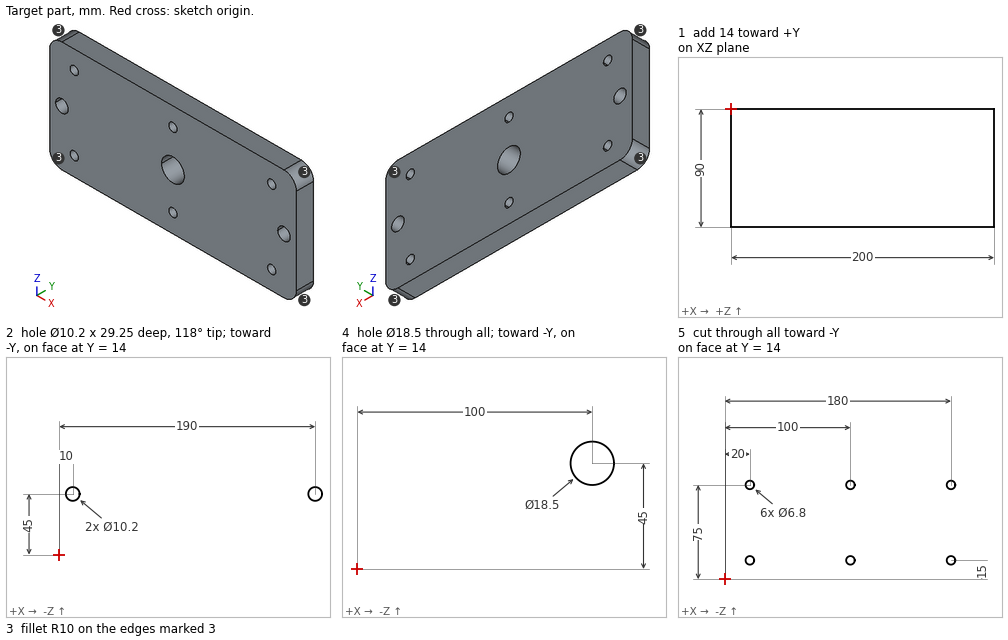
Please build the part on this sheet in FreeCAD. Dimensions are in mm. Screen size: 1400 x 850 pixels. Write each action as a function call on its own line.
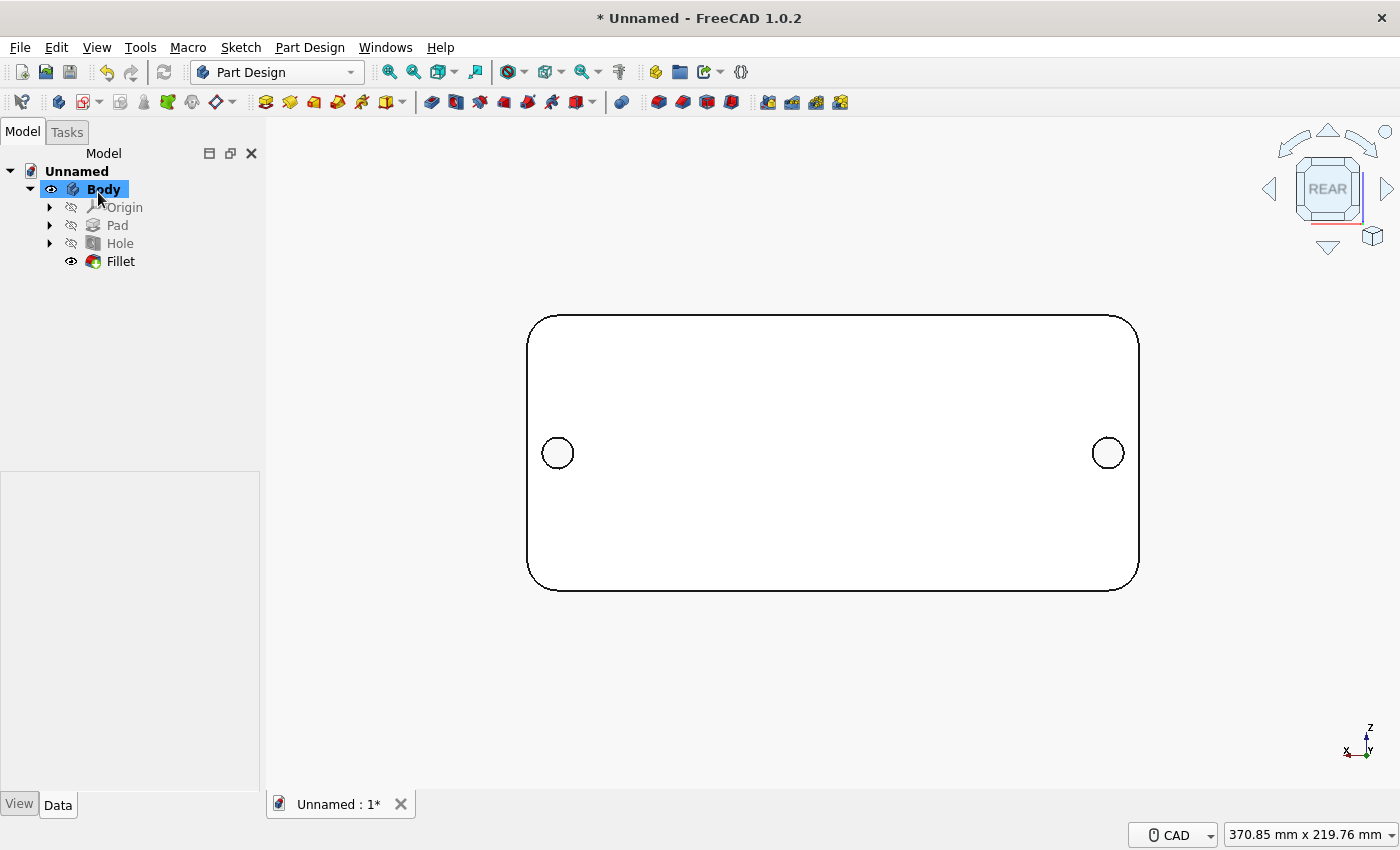
click(746, 452)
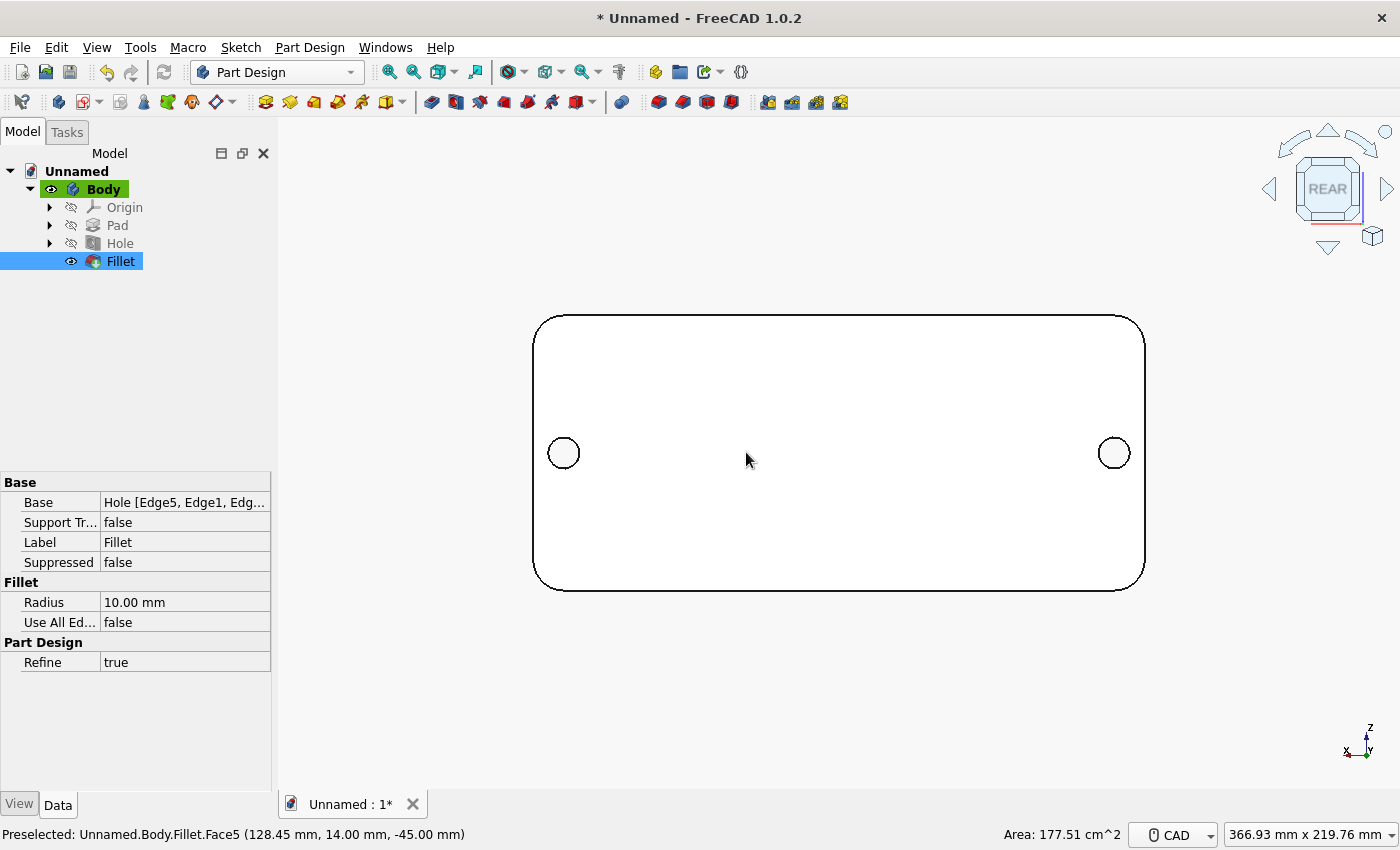
click(84, 102)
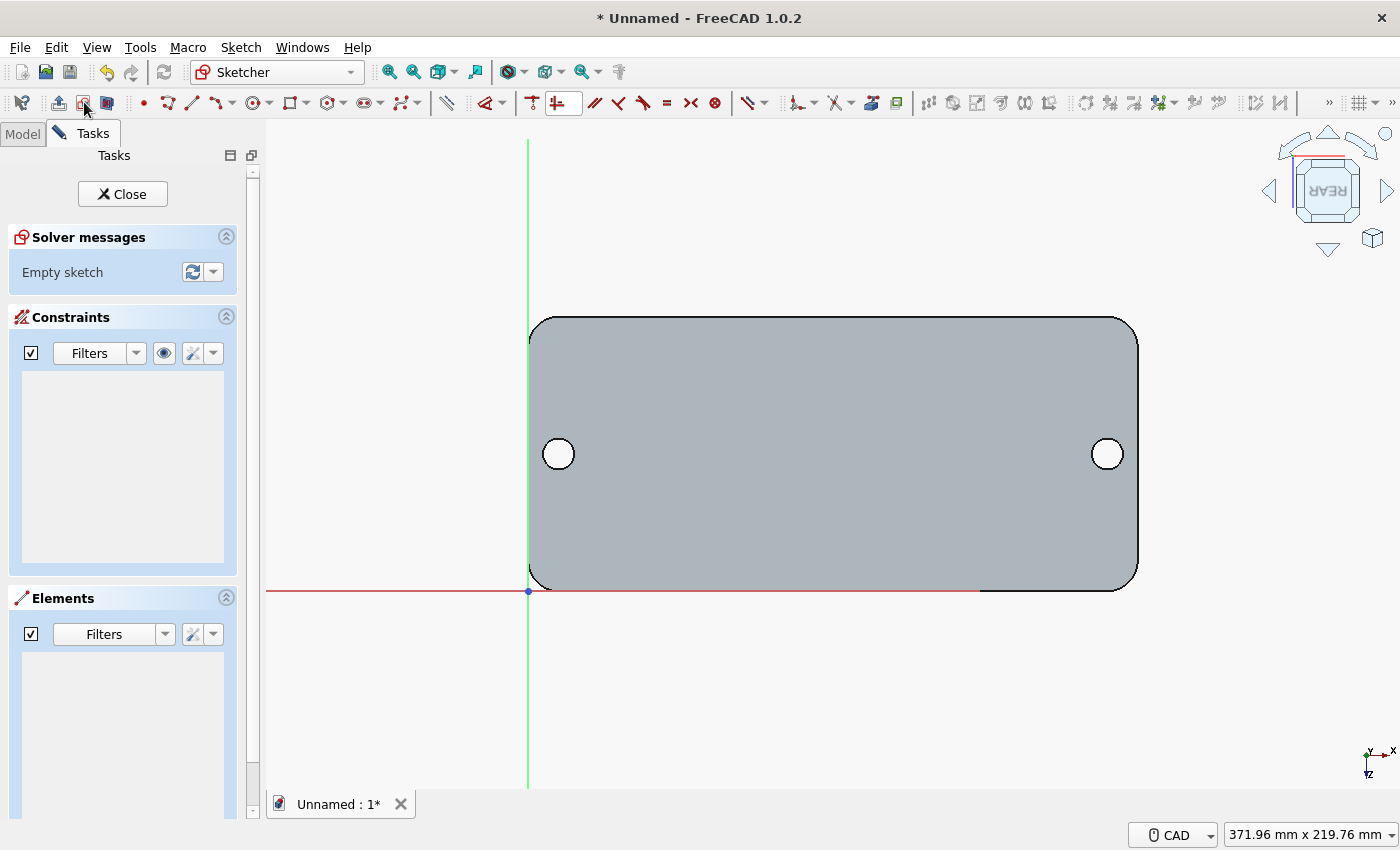
scroll(844, 454, up, 10)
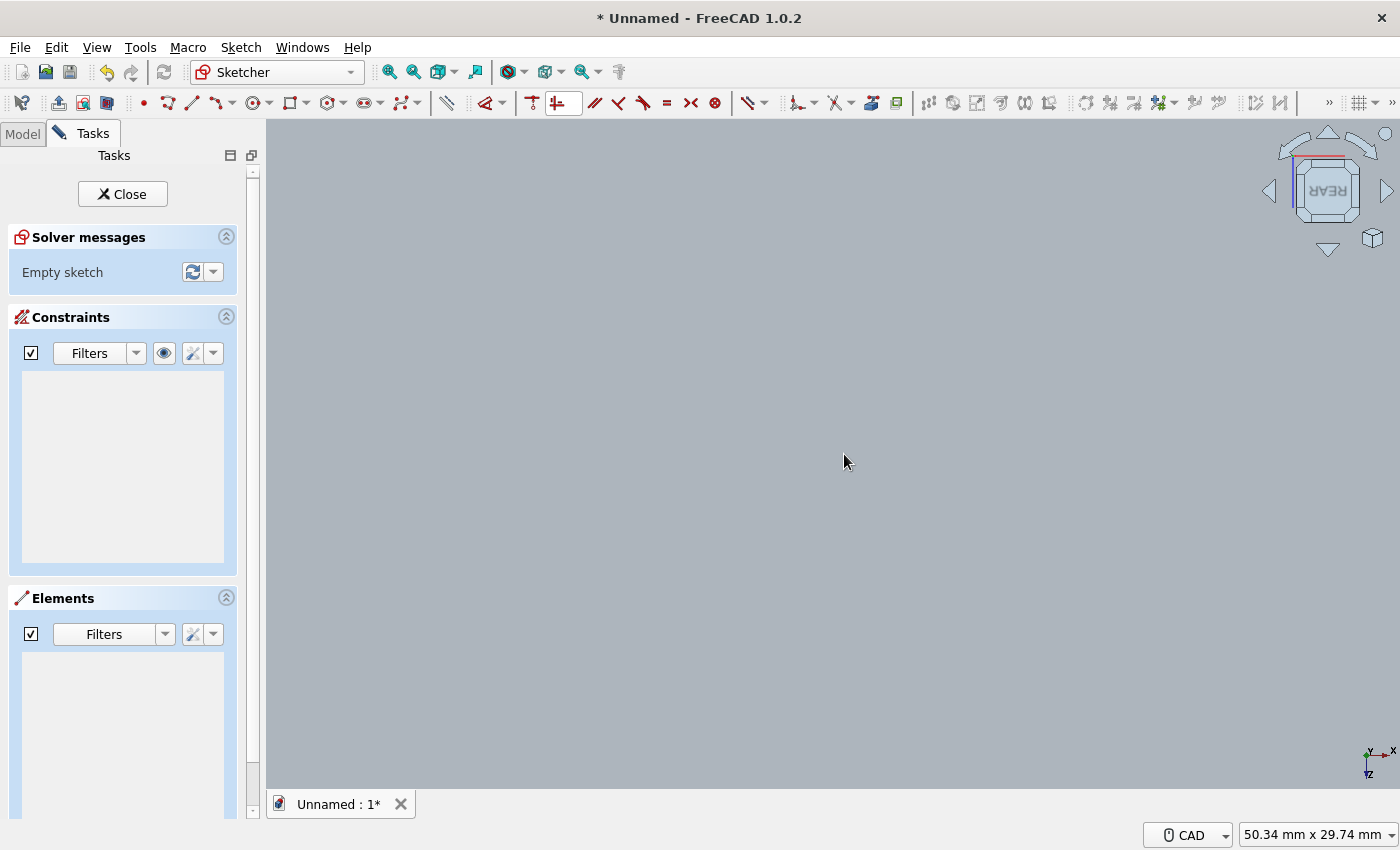
click(254, 104)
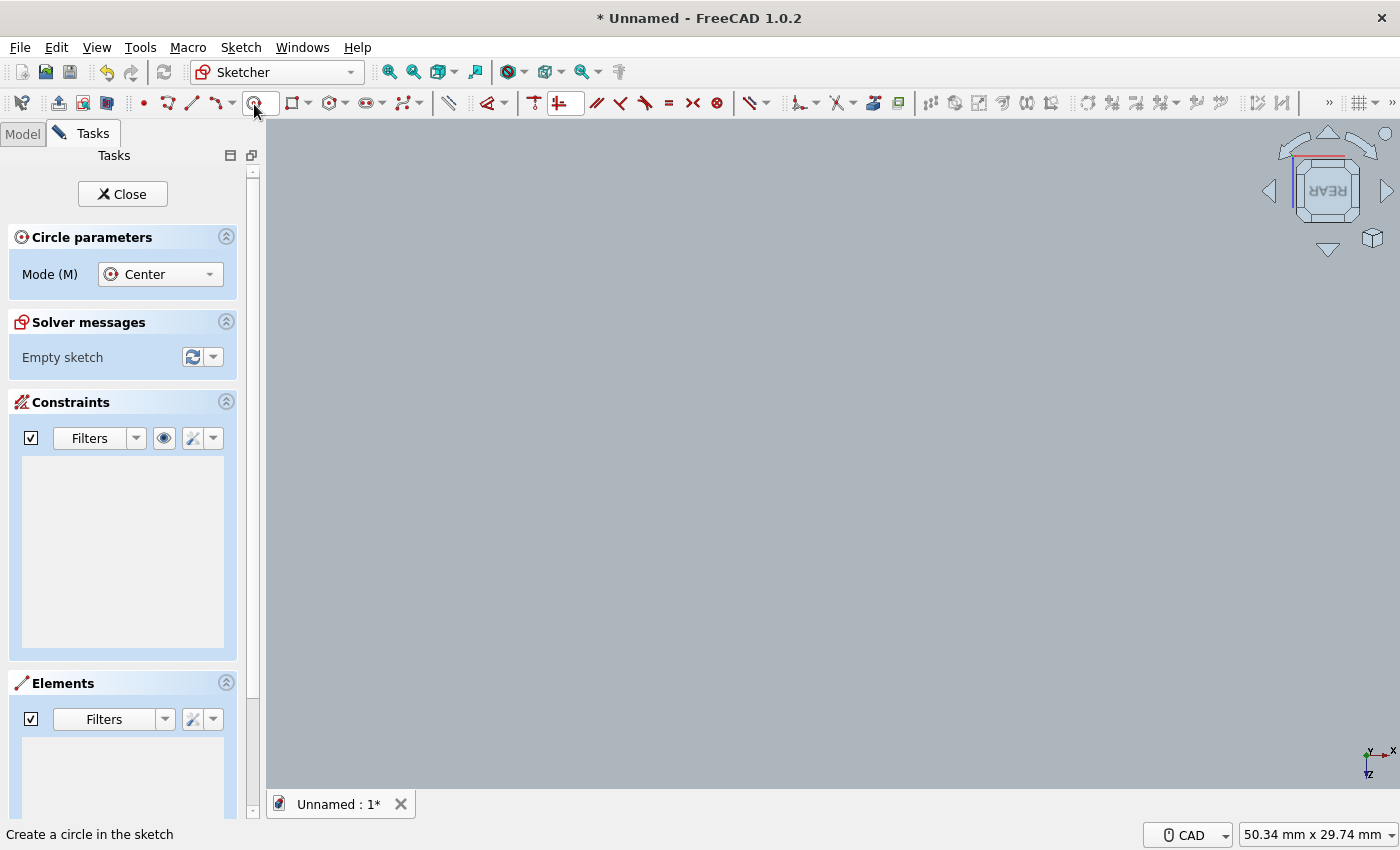
click(759, 451)
click(907, 303)
key(Escape)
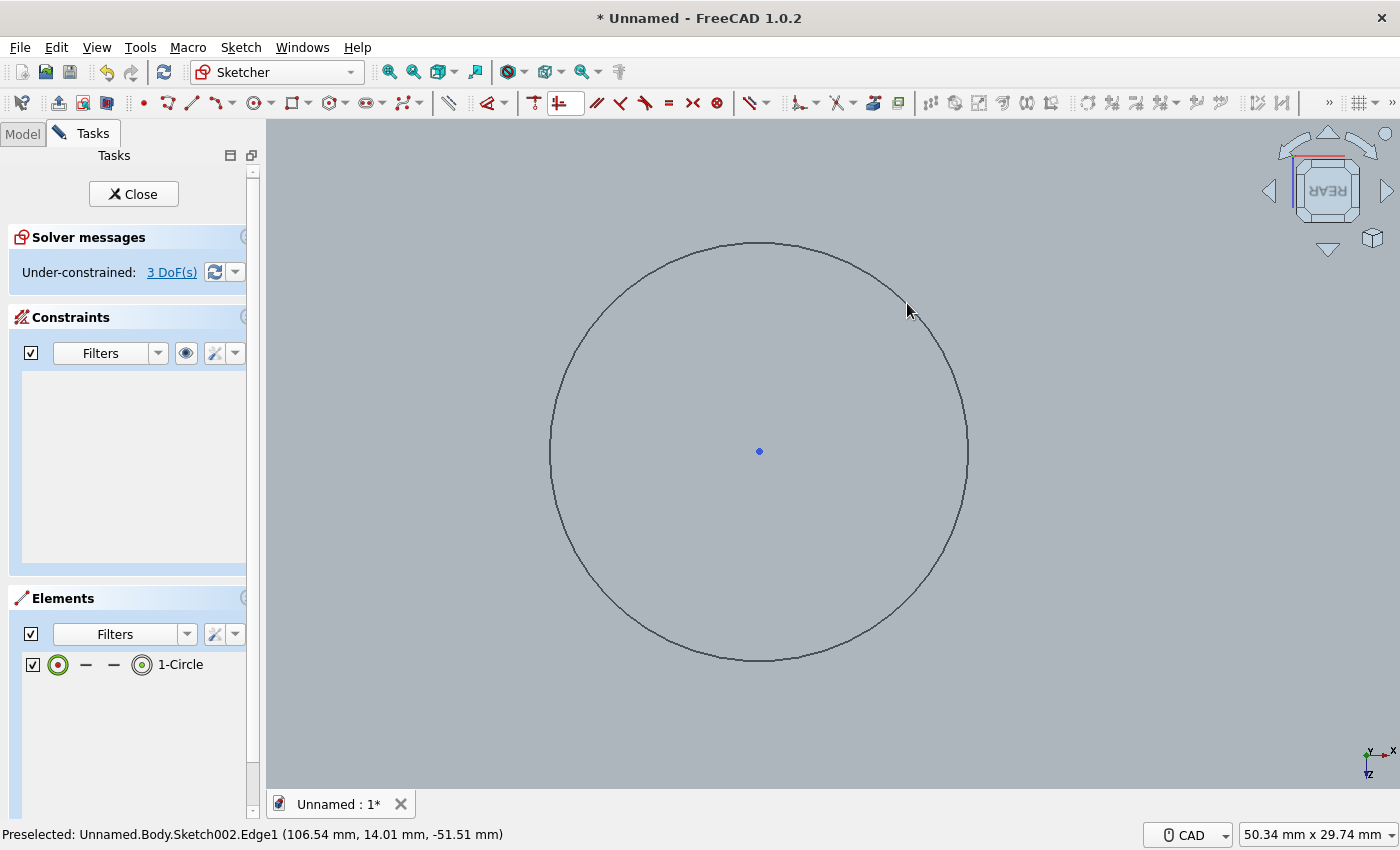
click(488, 104)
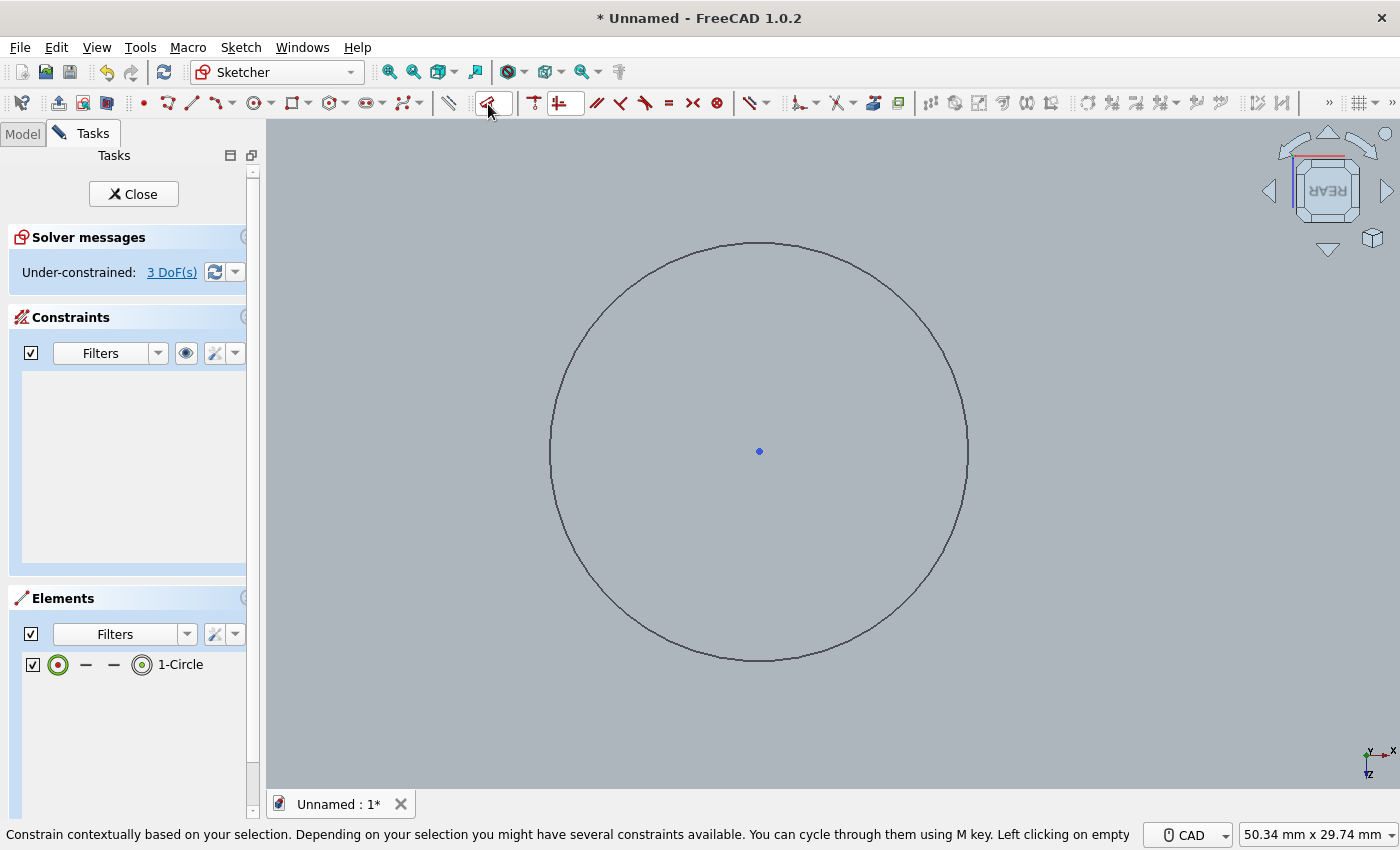
click(907, 304)
click(930, 281)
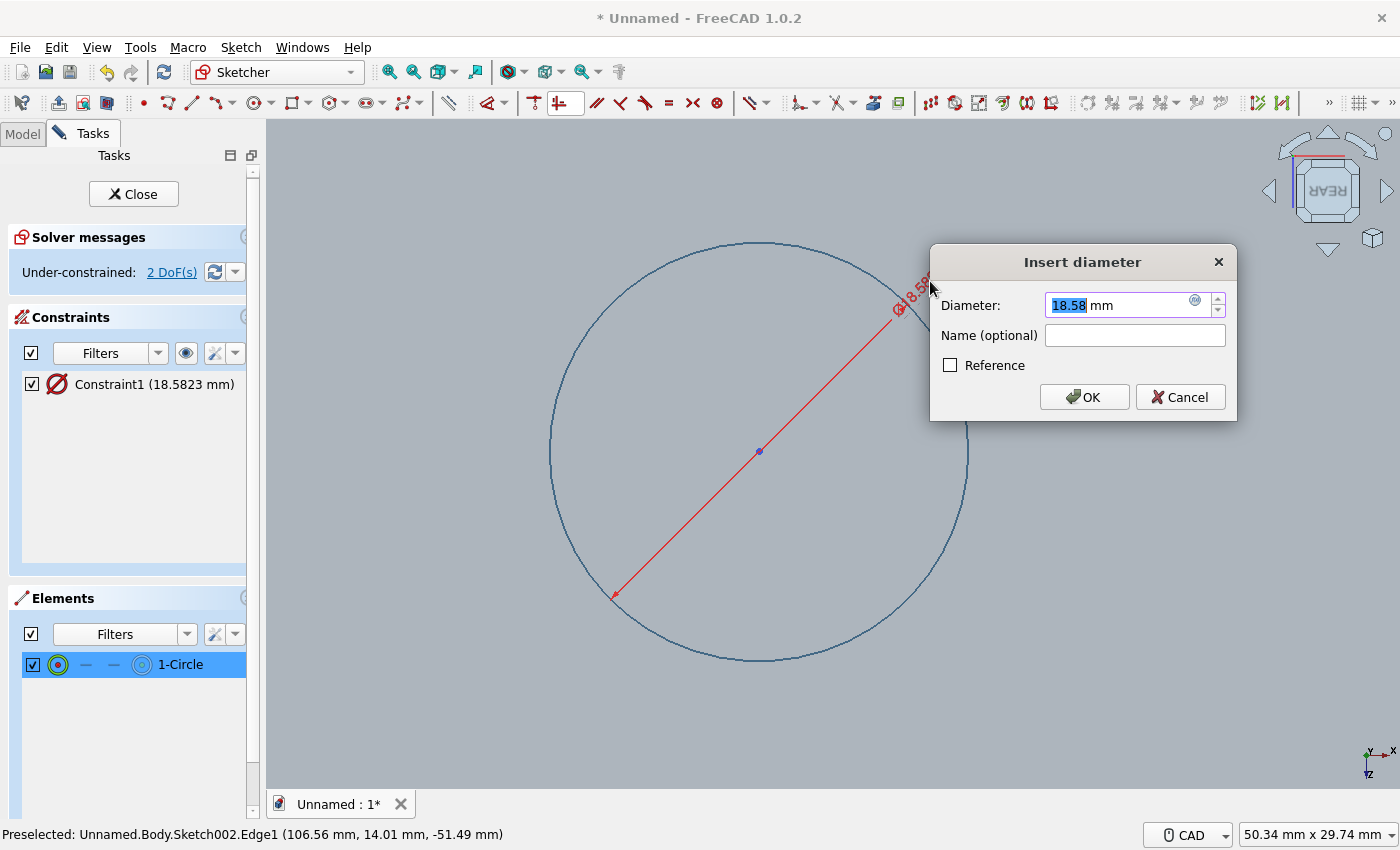
text(18.5)
key(Return)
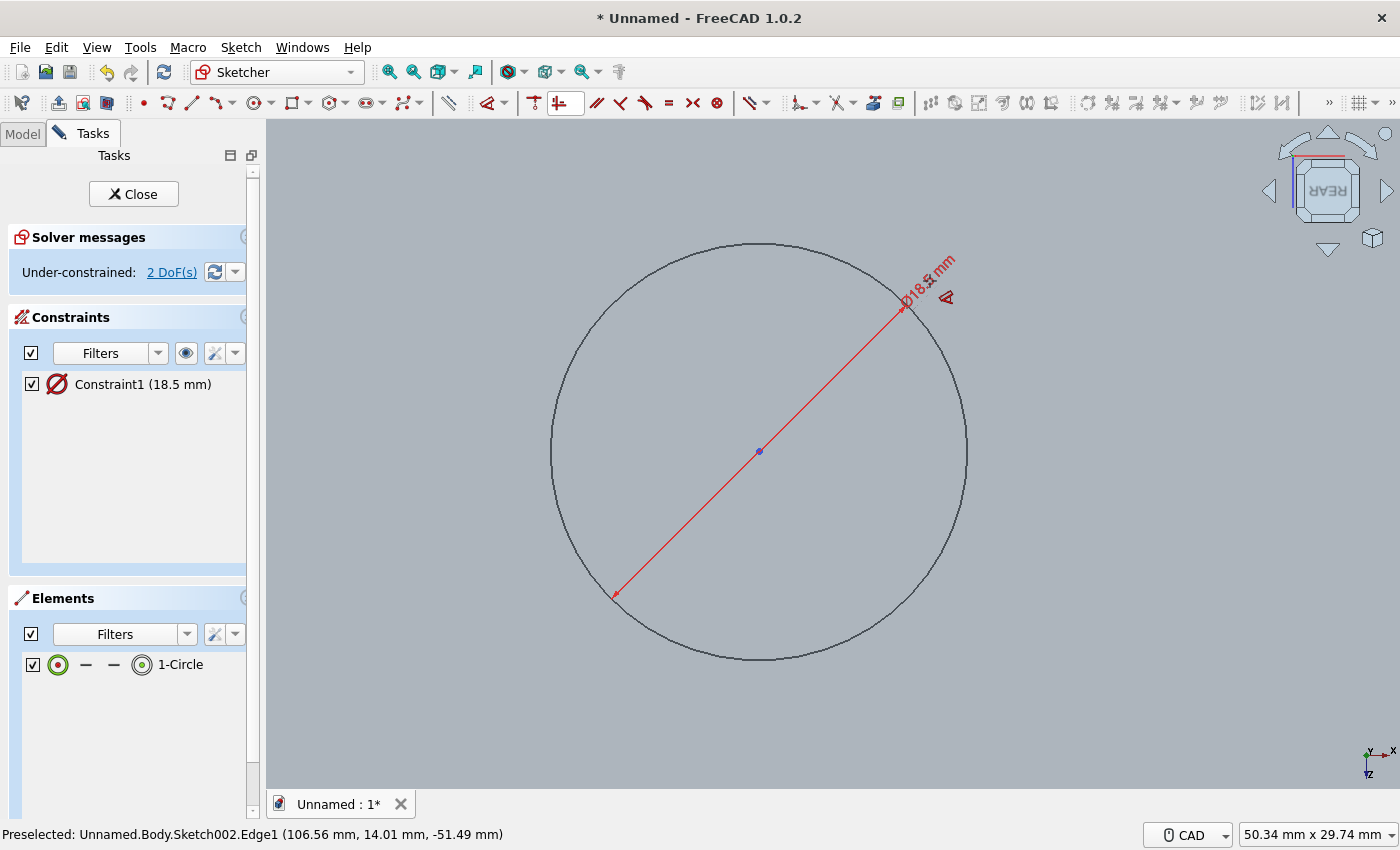
click(759, 452)
click(793, 607)